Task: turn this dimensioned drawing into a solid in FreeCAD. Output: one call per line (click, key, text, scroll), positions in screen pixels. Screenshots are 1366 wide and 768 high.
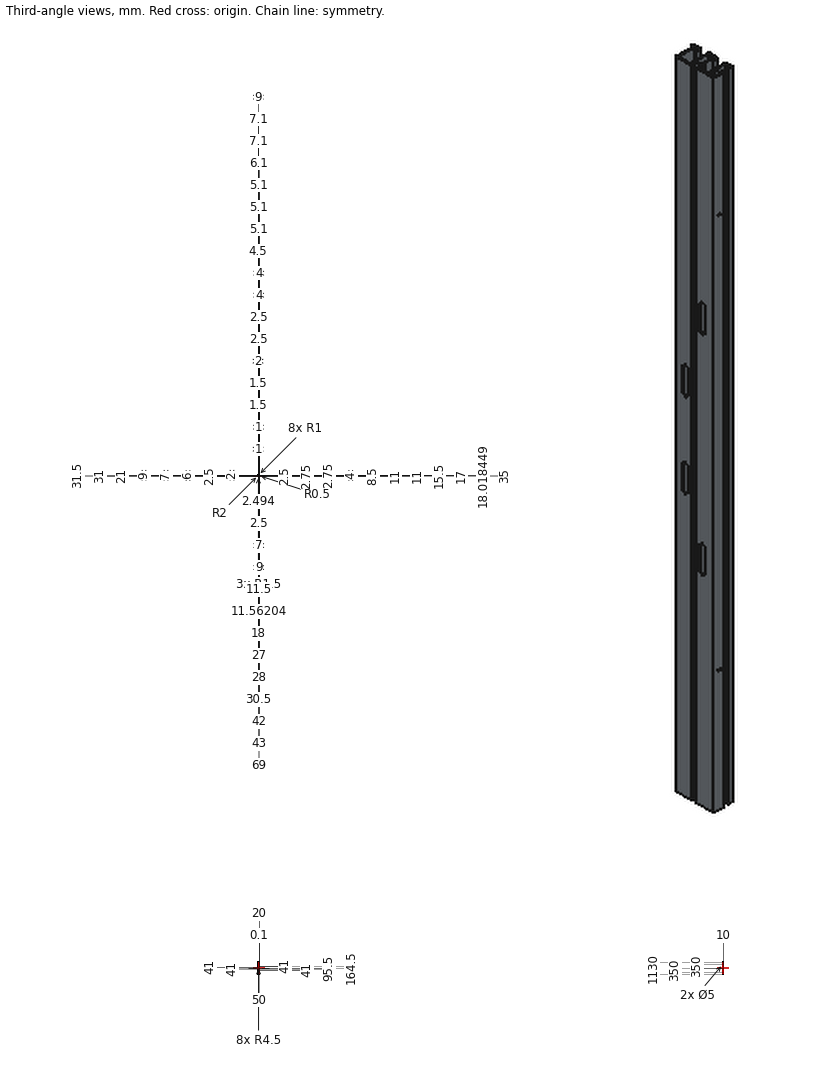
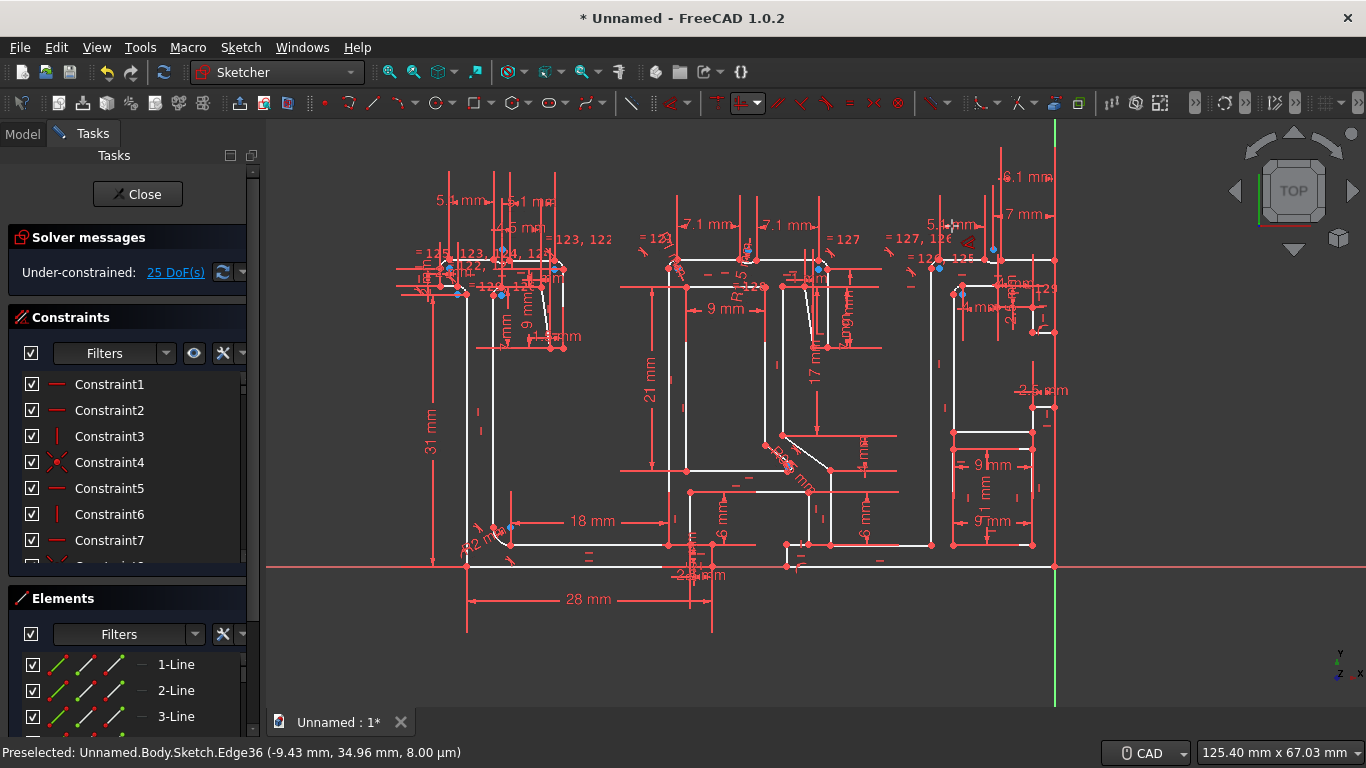
click(831, 523)
click(865, 491)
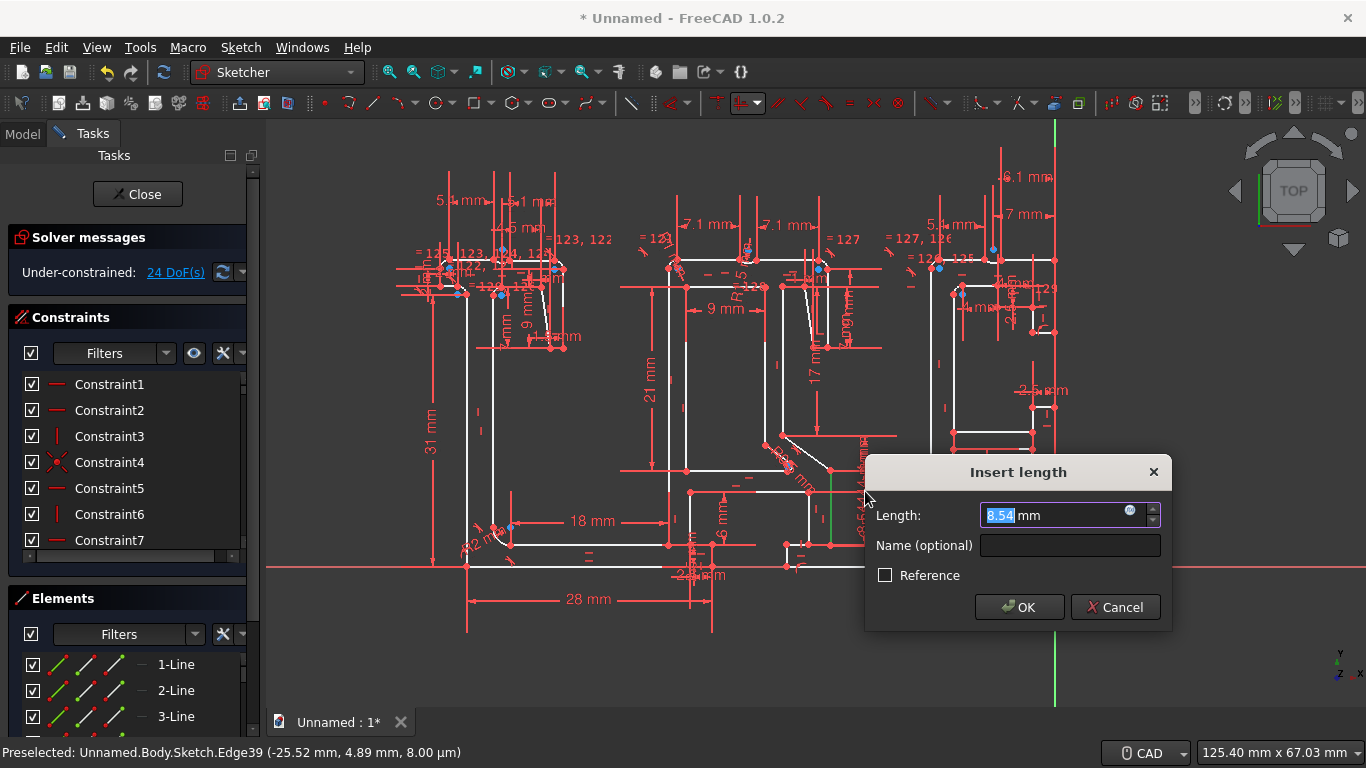
text(8.5)
key(Return)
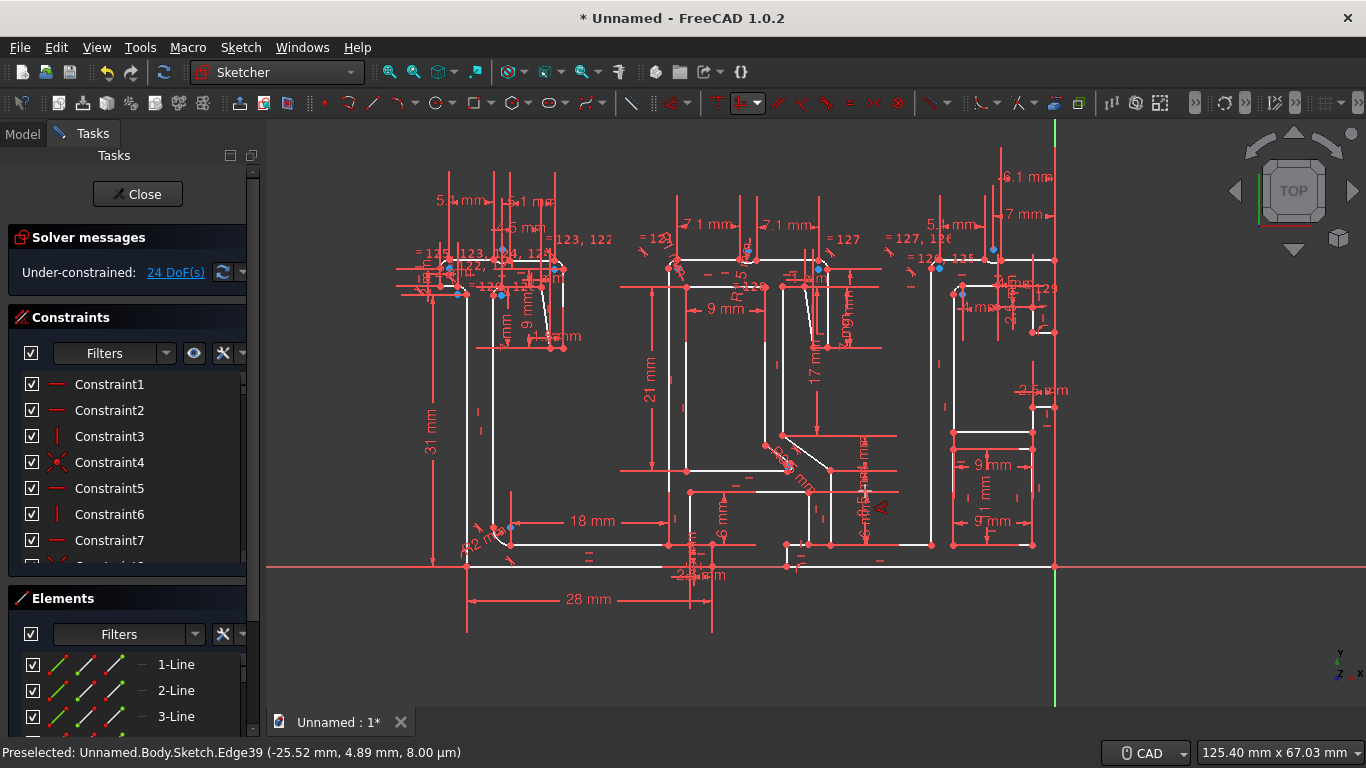
scroll(794, 287, up, 3)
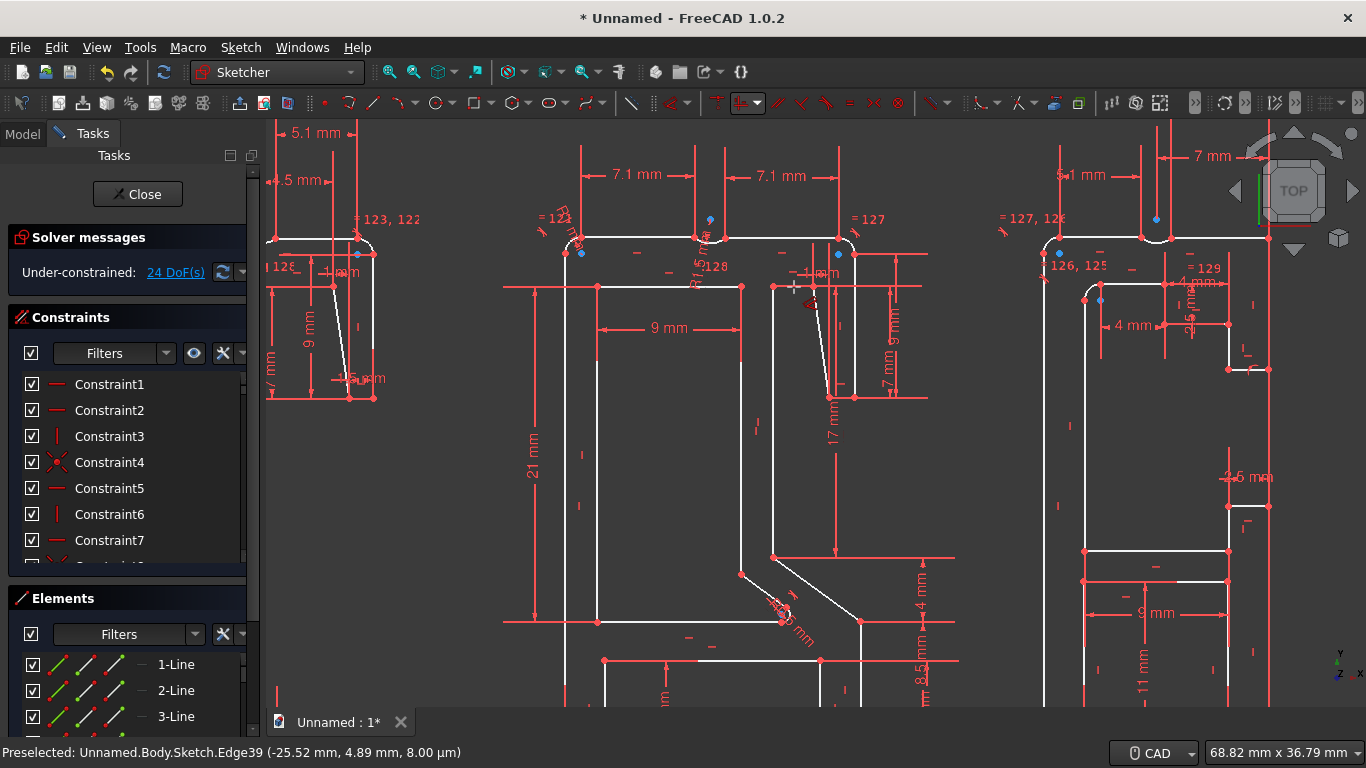
click(793, 286)
click(793, 252)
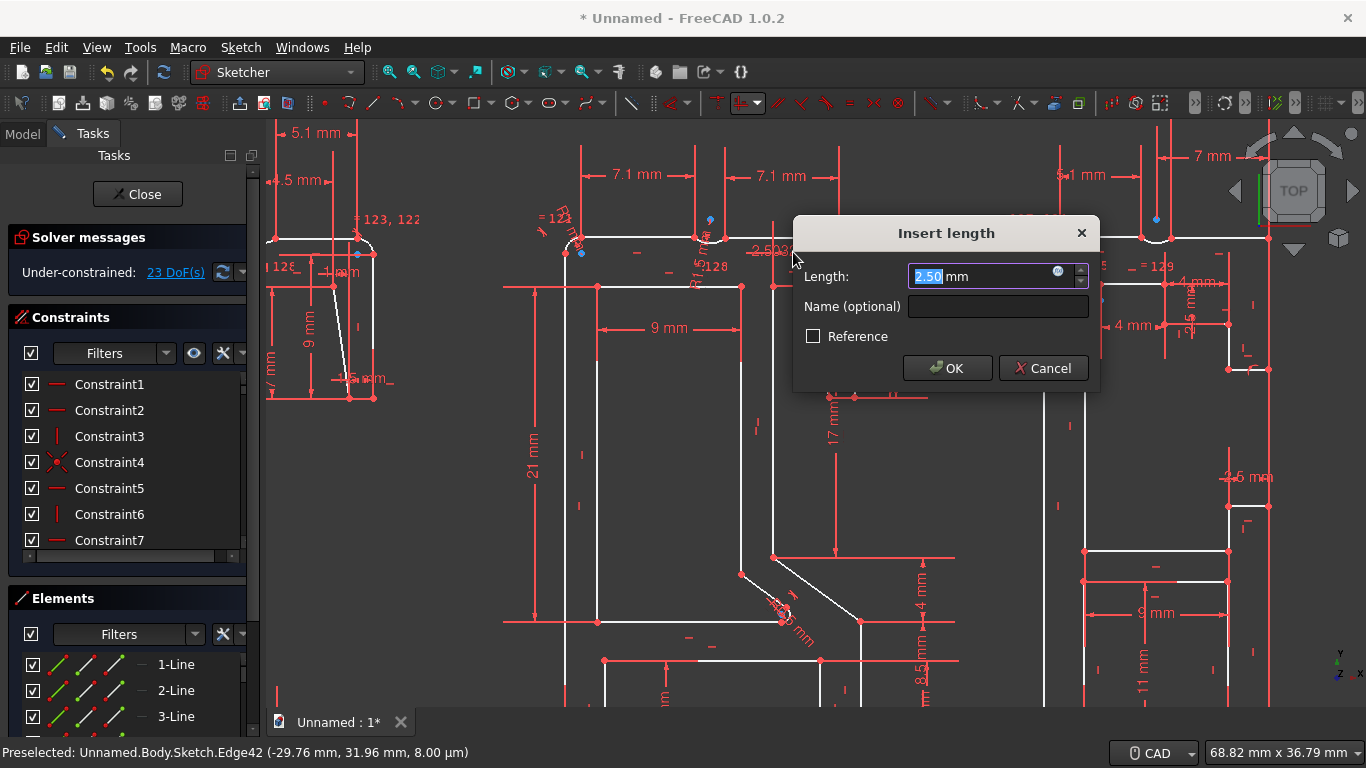
text(2.5)
key(Return)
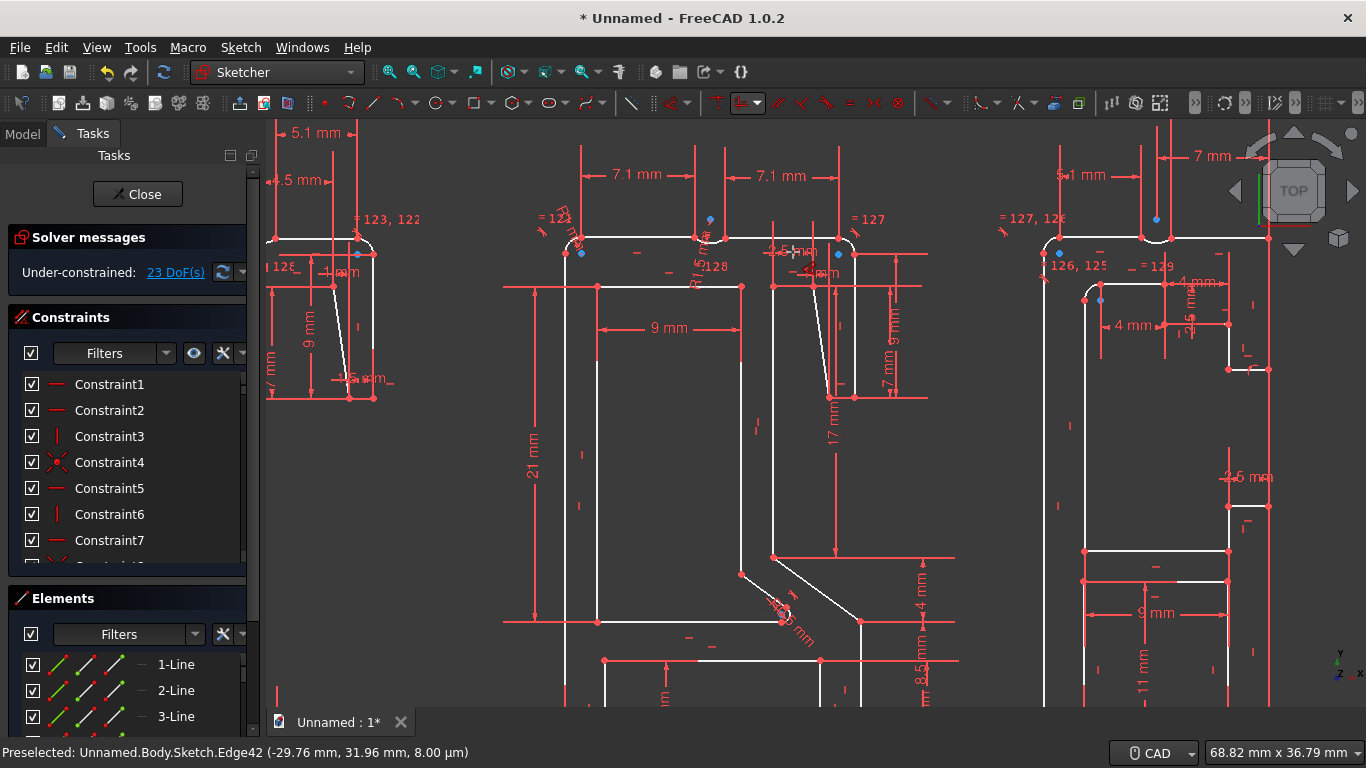
scroll(839, 398, up, 3)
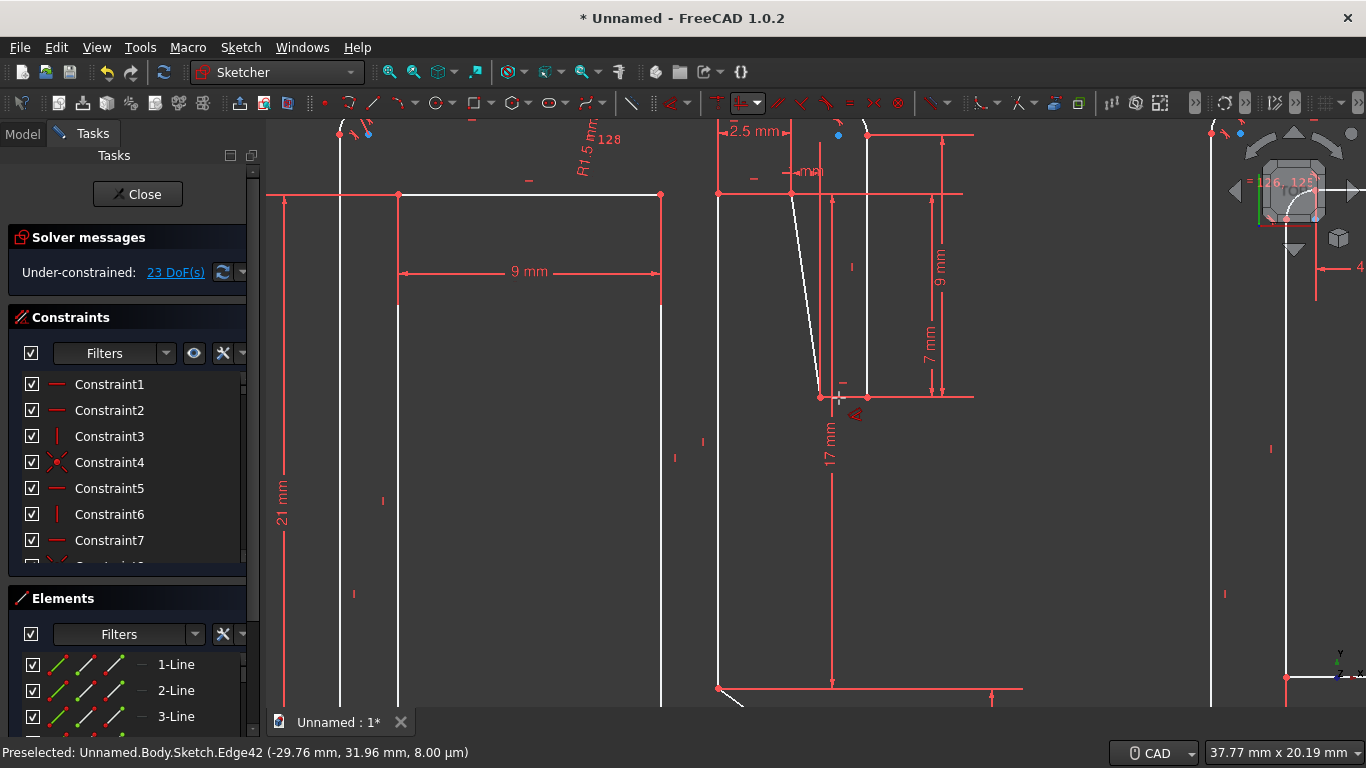
click(839, 397)
click(844, 363)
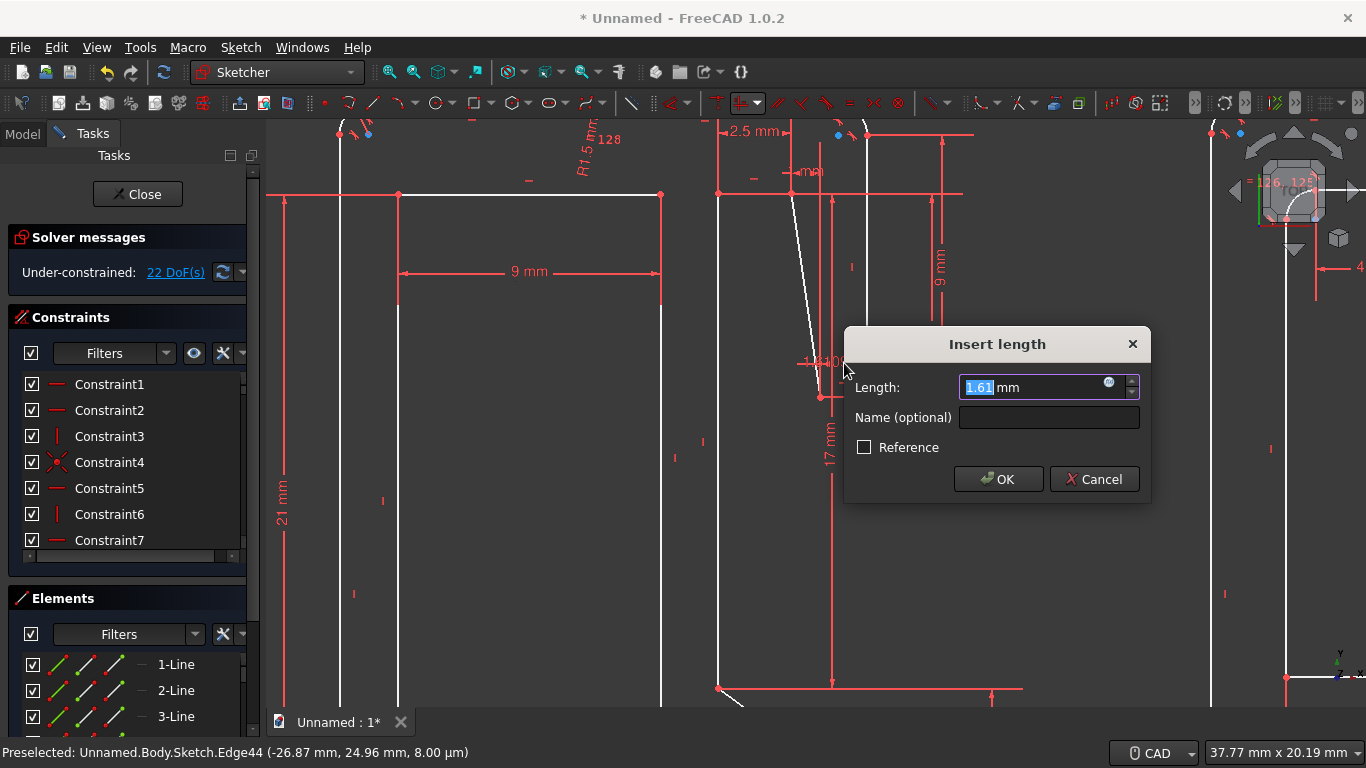
text(1.5)
key(Return)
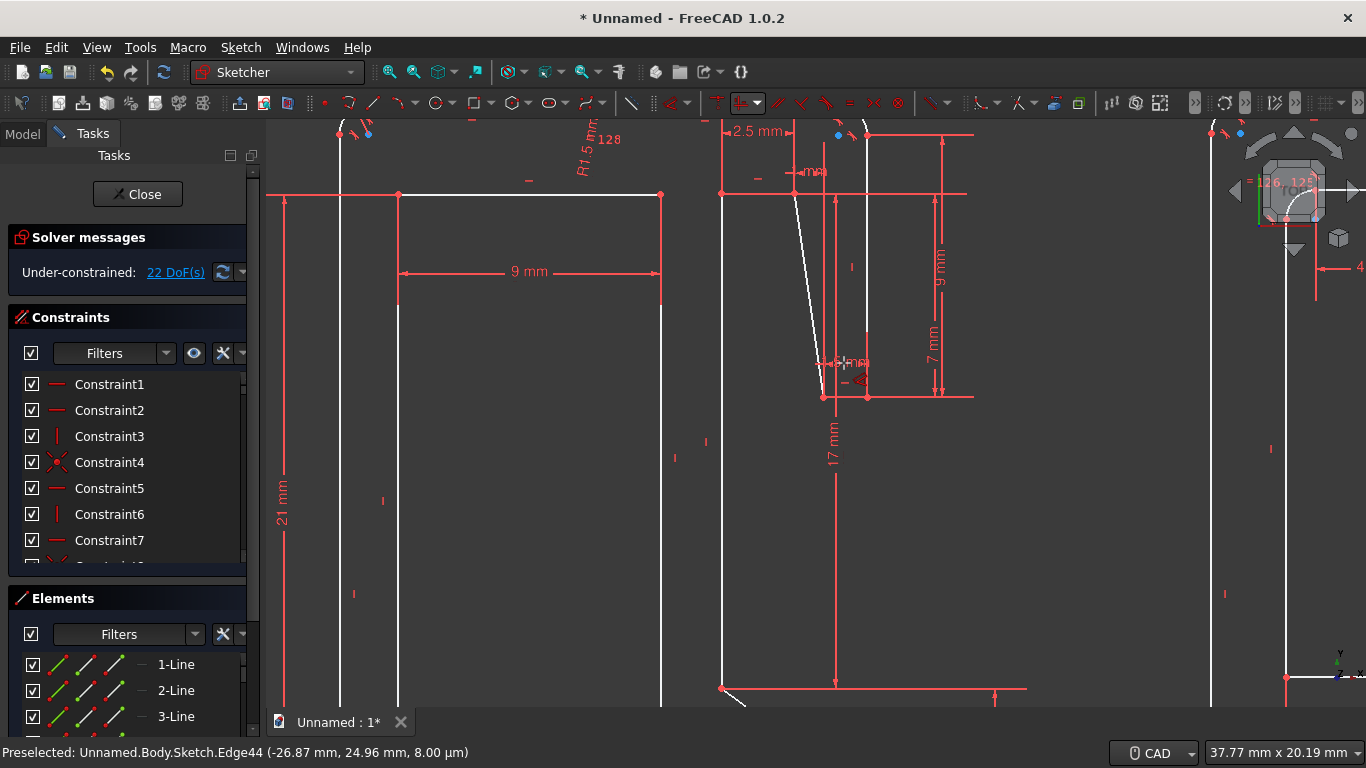
scroll(810, 326, down, 6)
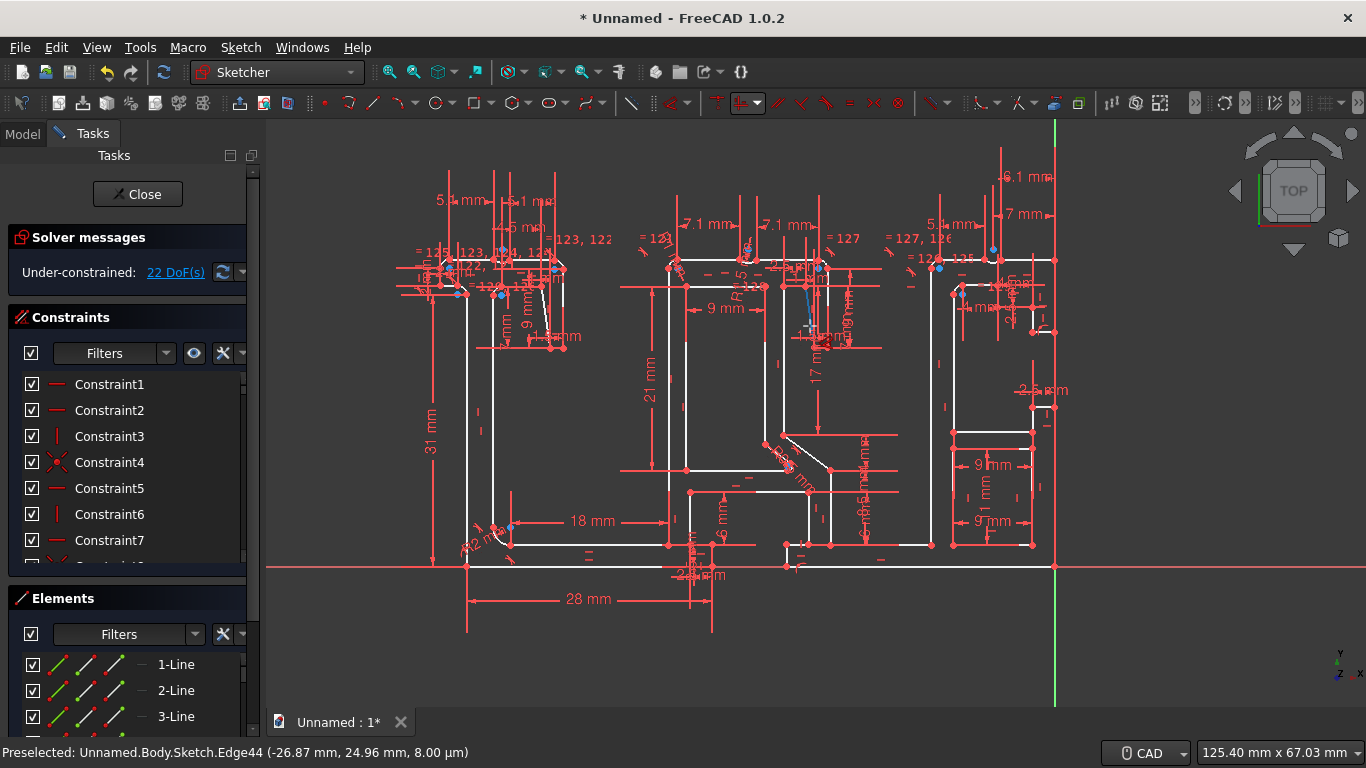
scroll(819, 260, up, 2)